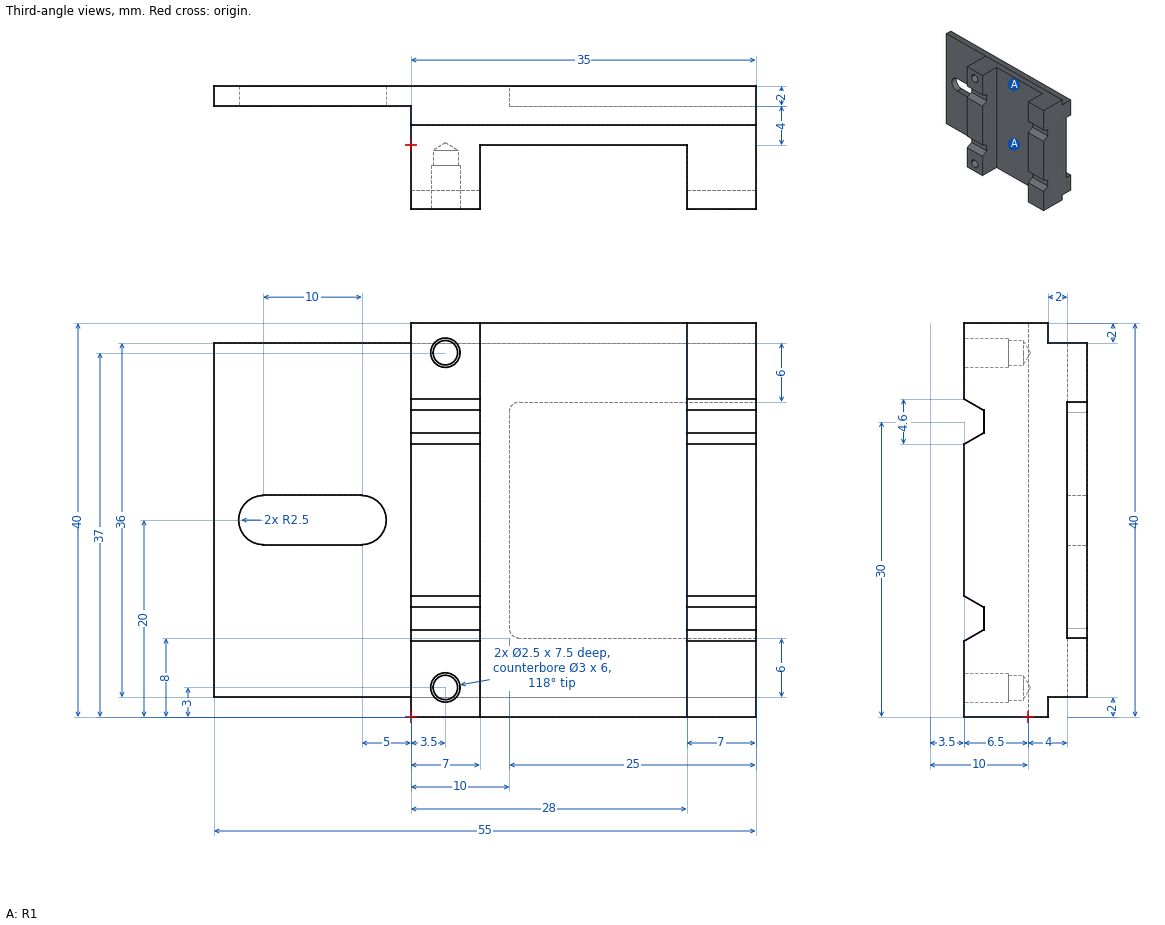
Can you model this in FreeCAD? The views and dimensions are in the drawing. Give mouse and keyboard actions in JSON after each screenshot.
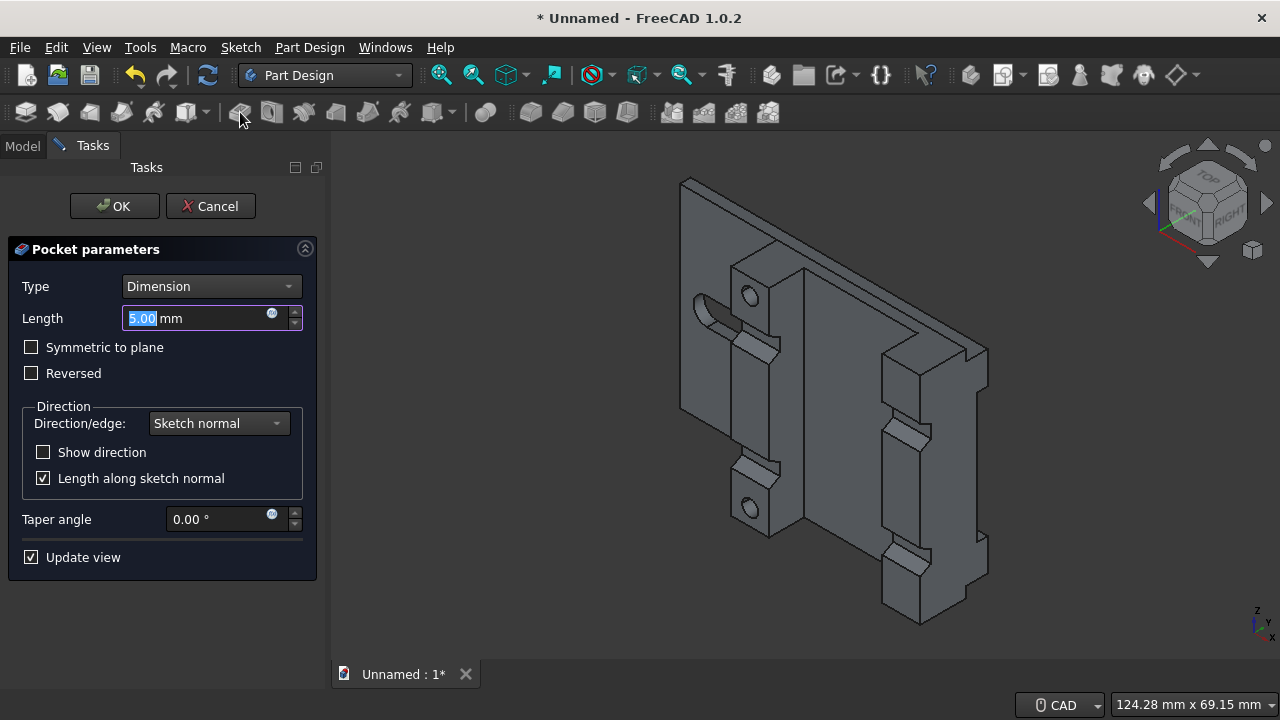
{"action": "left_click", "coordinate": [212, 286]}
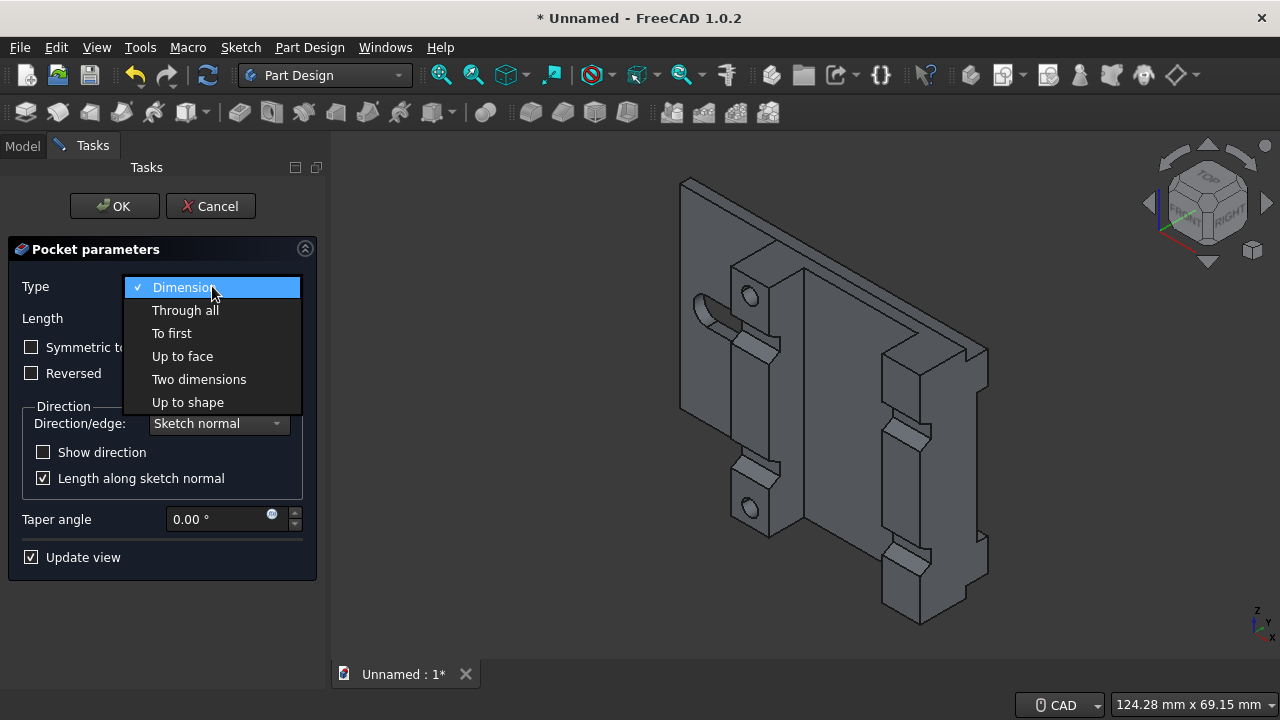
{"action": "left_click", "coordinate": [212, 310]}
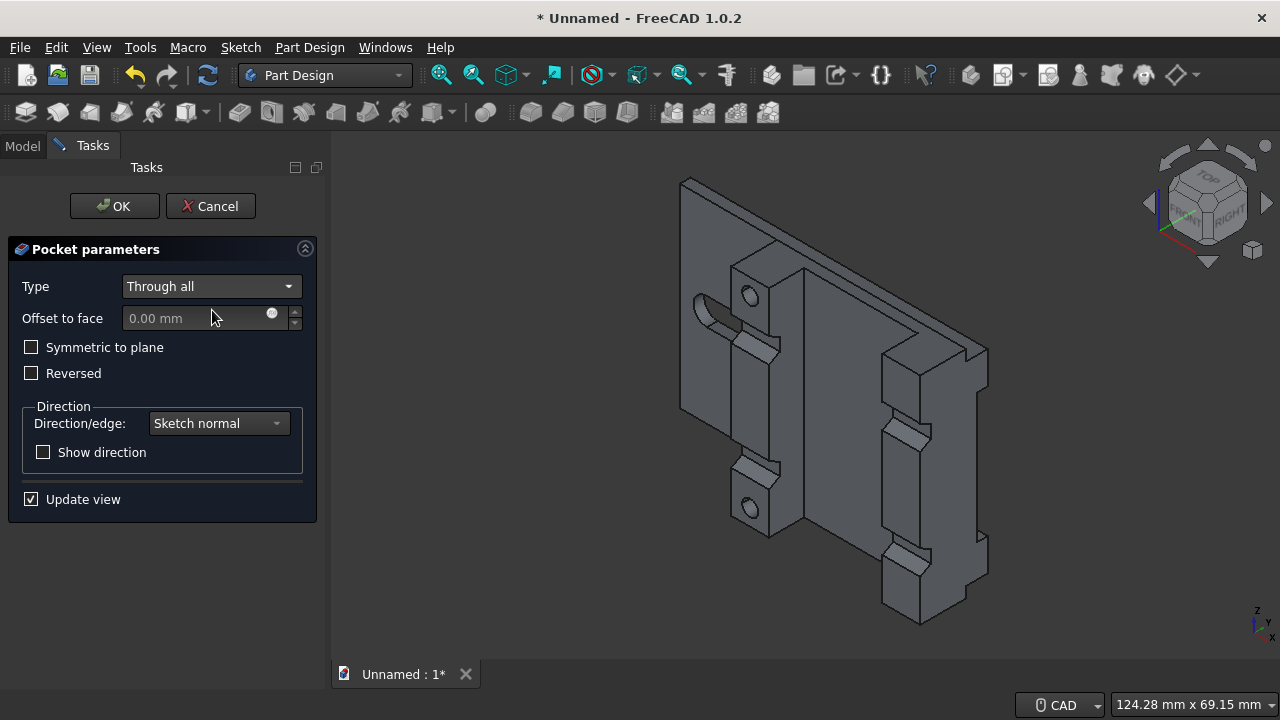
{"action": "left_click", "coordinate": [115, 206]}